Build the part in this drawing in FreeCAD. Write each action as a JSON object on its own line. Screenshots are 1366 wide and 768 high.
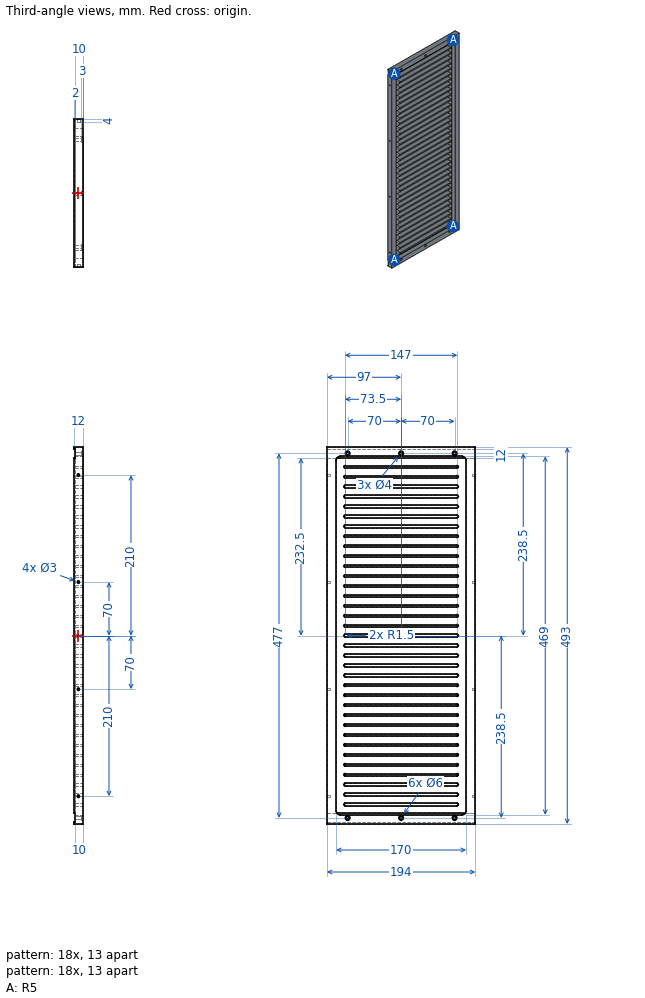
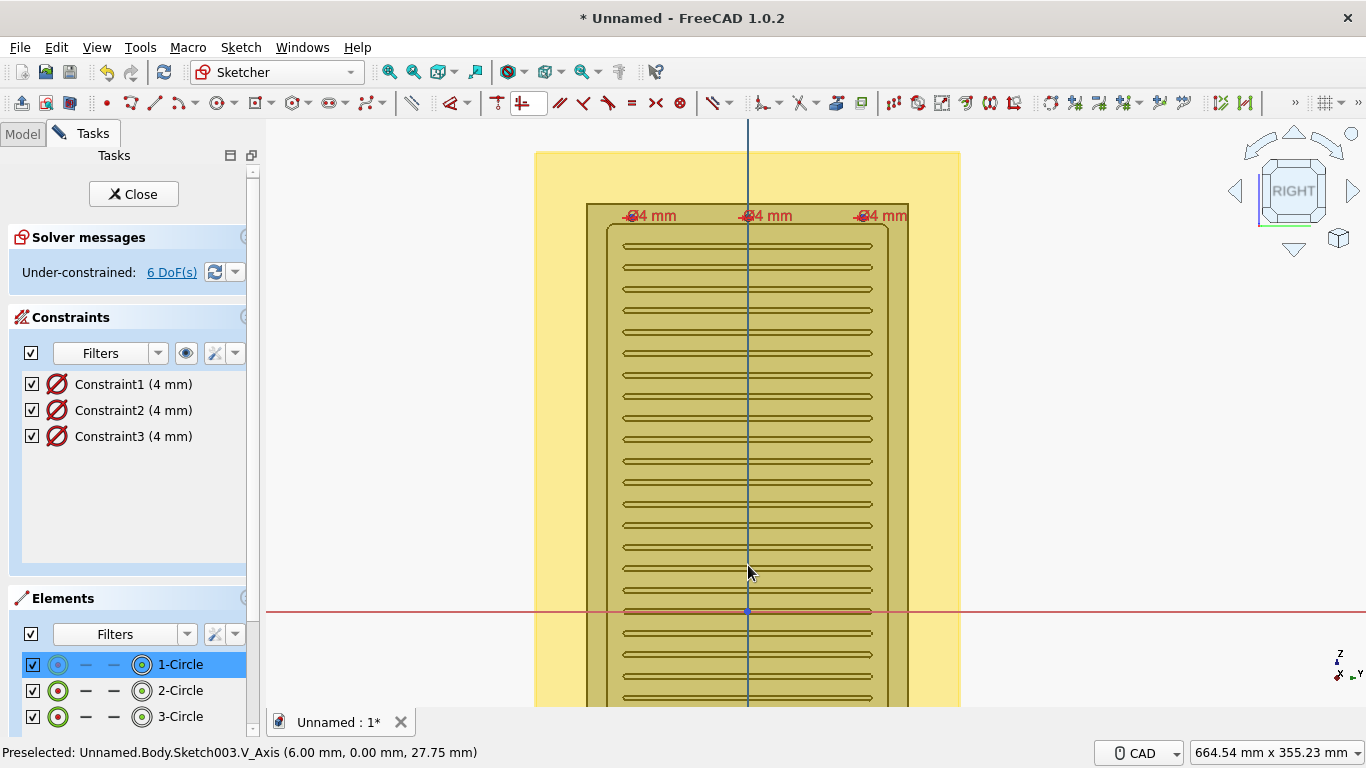
{"action": "left_click", "coordinate": [498, 104]}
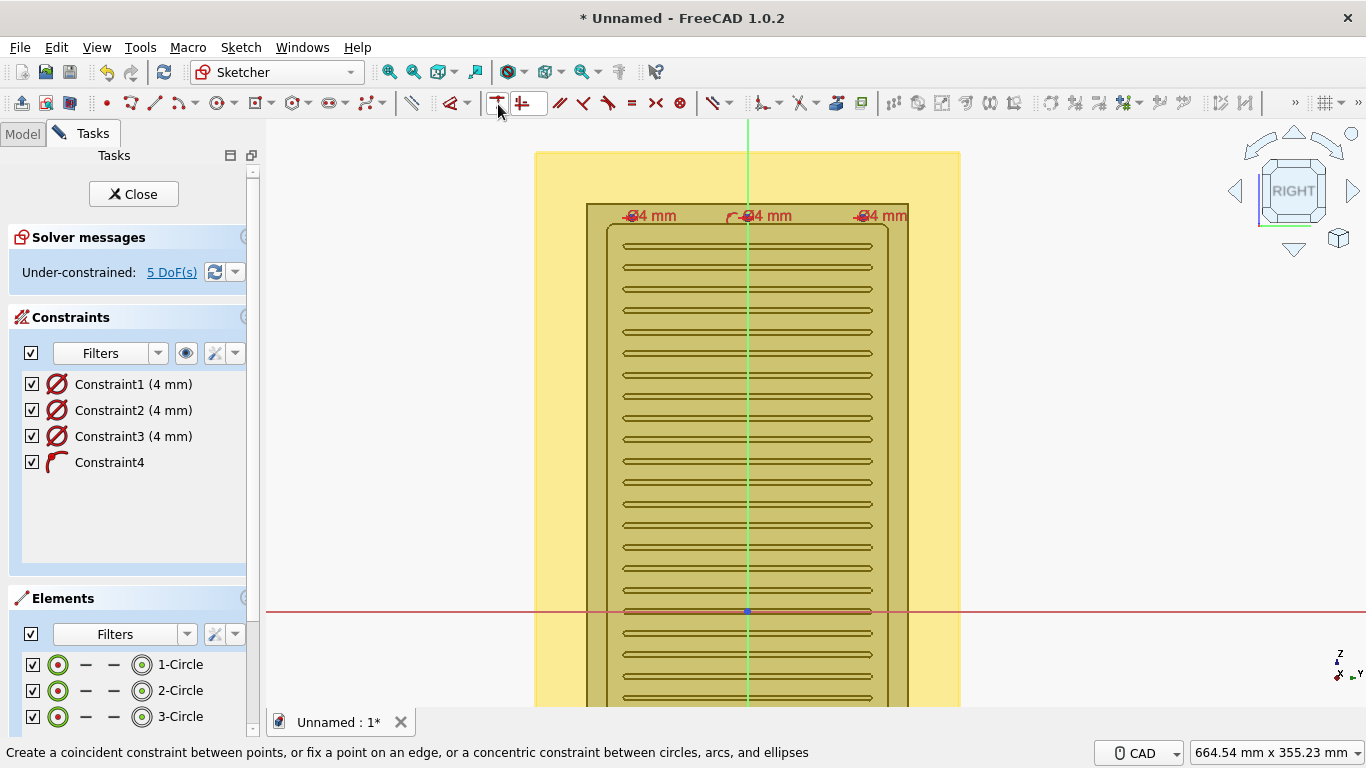
{"action": "left_click", "coordinate": [748, 218]}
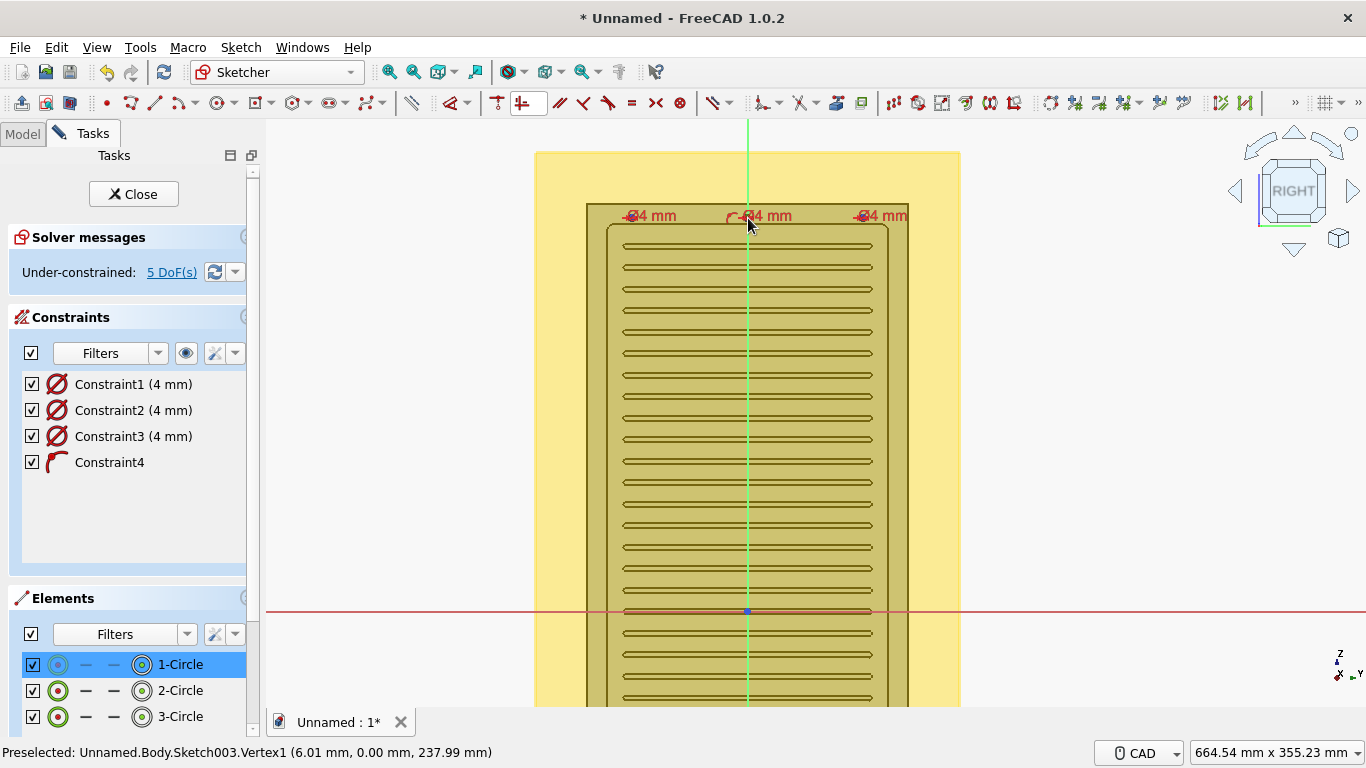
{"action": "left_click", "coordinate": [863, 218]}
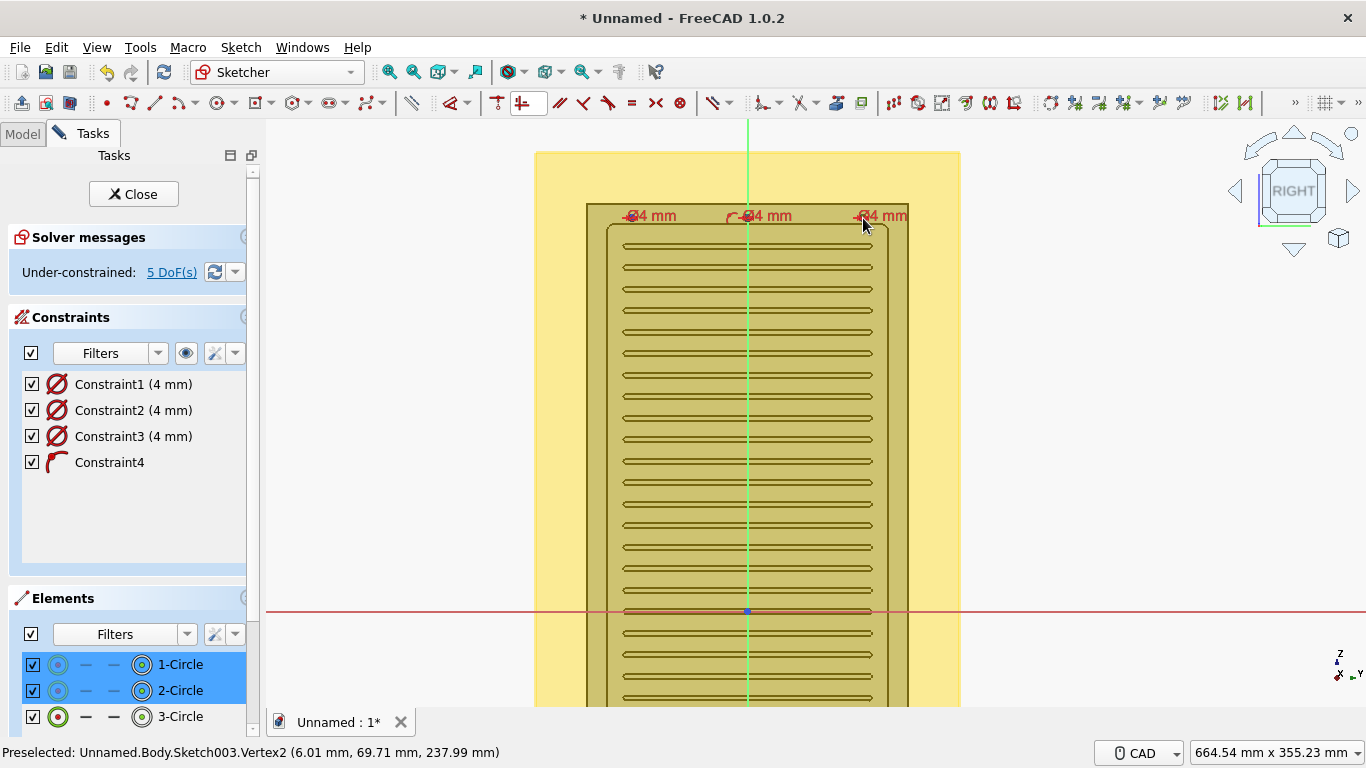
{"action": "left_click", "coordinate": [542, 104]}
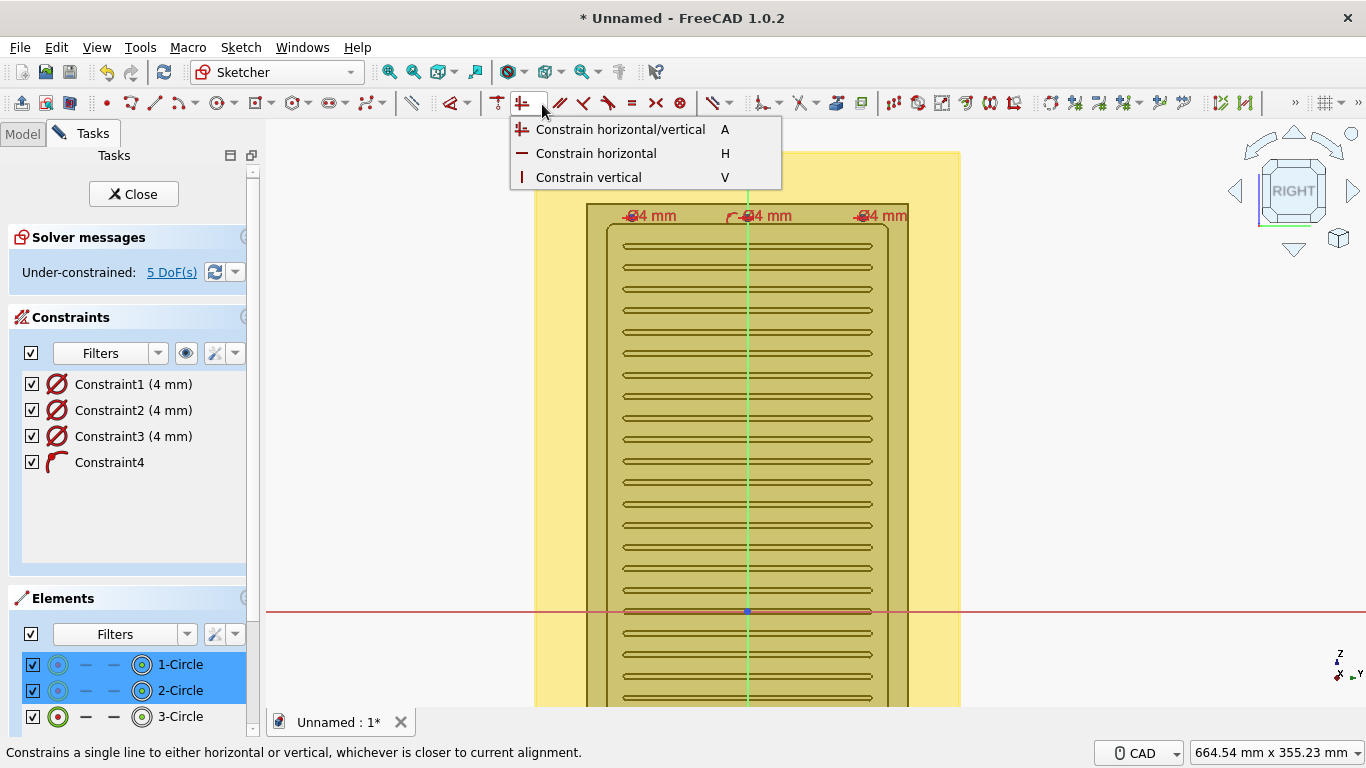
{"action": "left_click", "coordinate": [646, 153]}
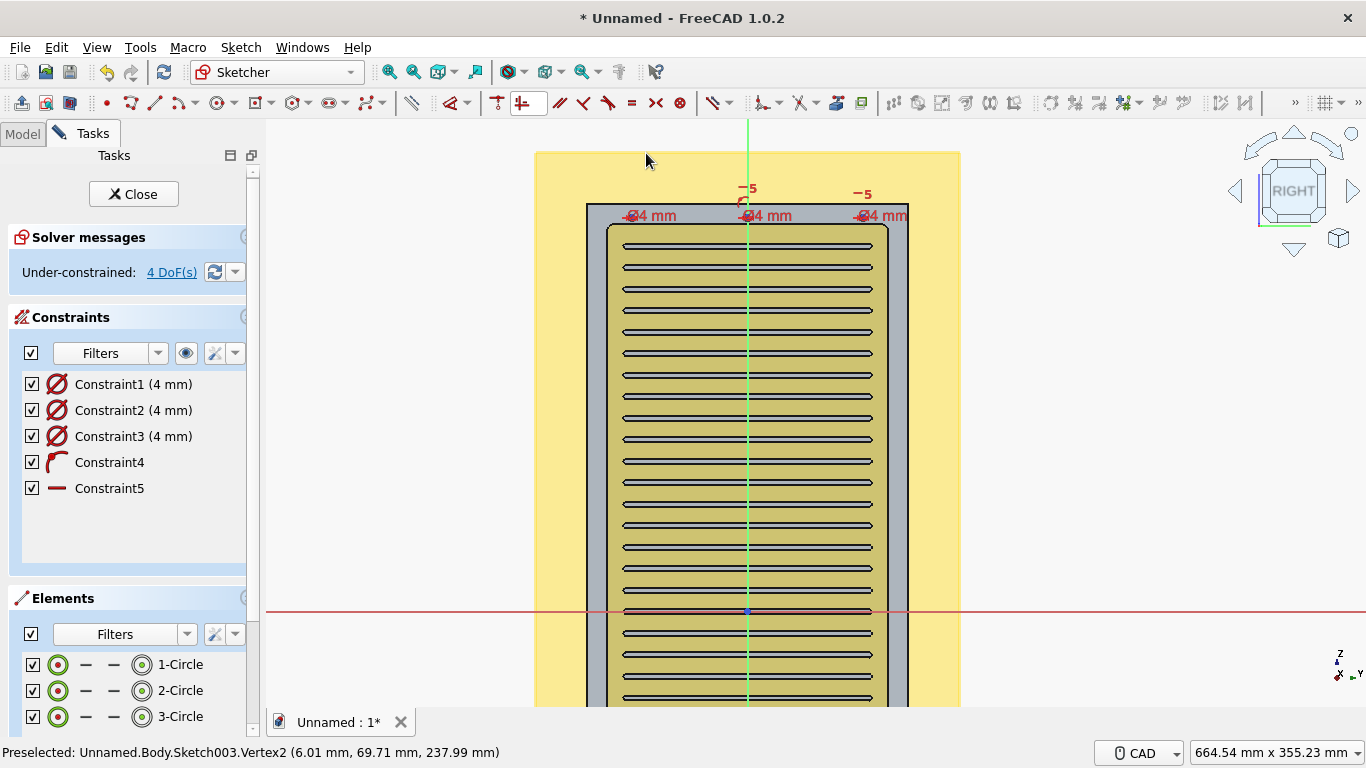
{"action": "left_click", "coordinate": [748, 218]}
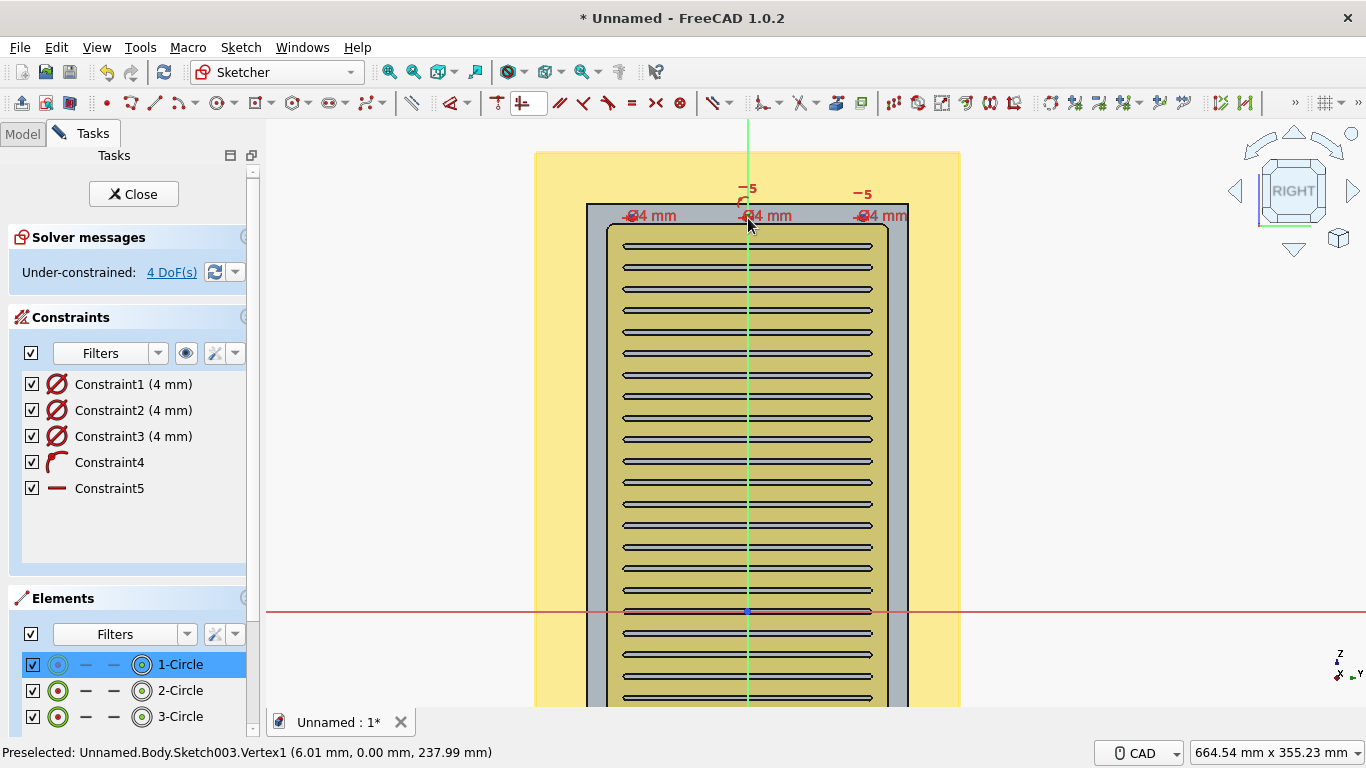
{"action": "left_click", "coordinate": [632, 218]}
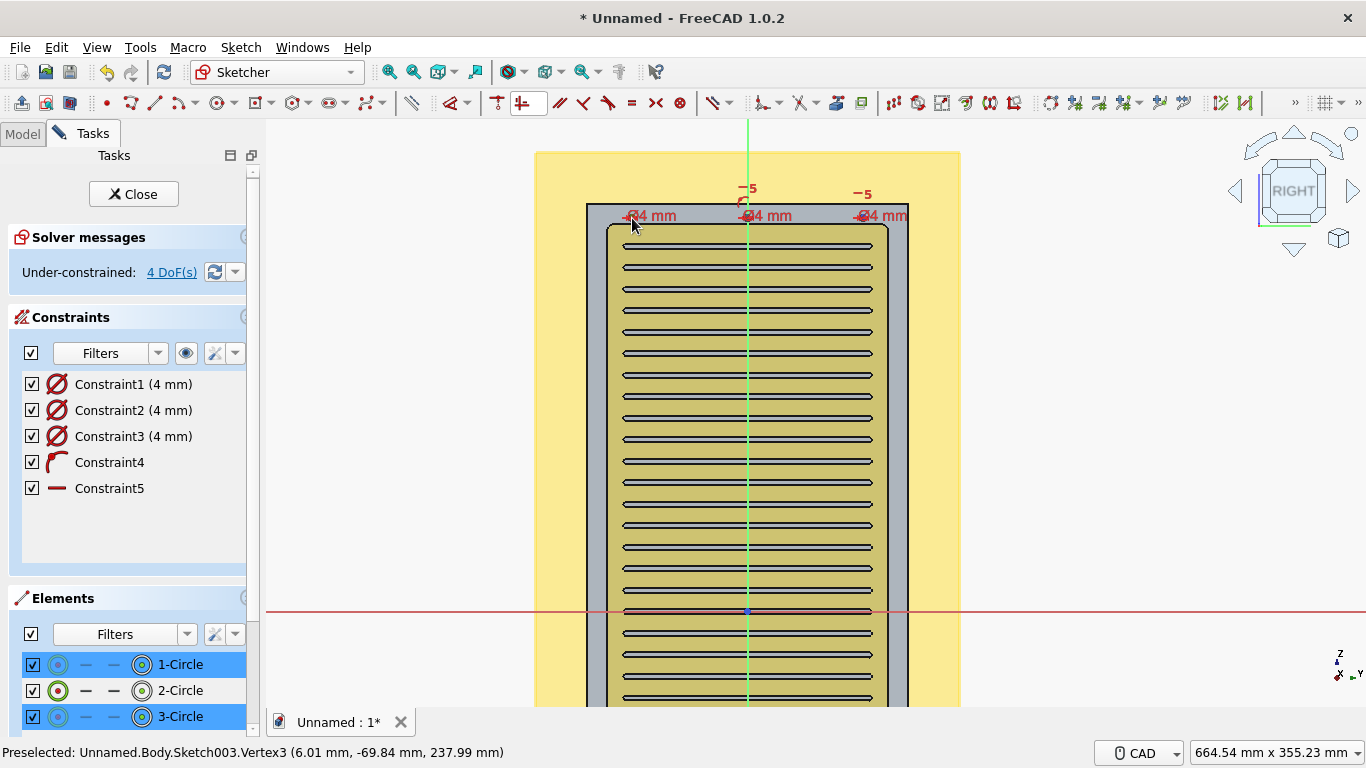
{"action": "left_click", "coordinate": [542, 104]}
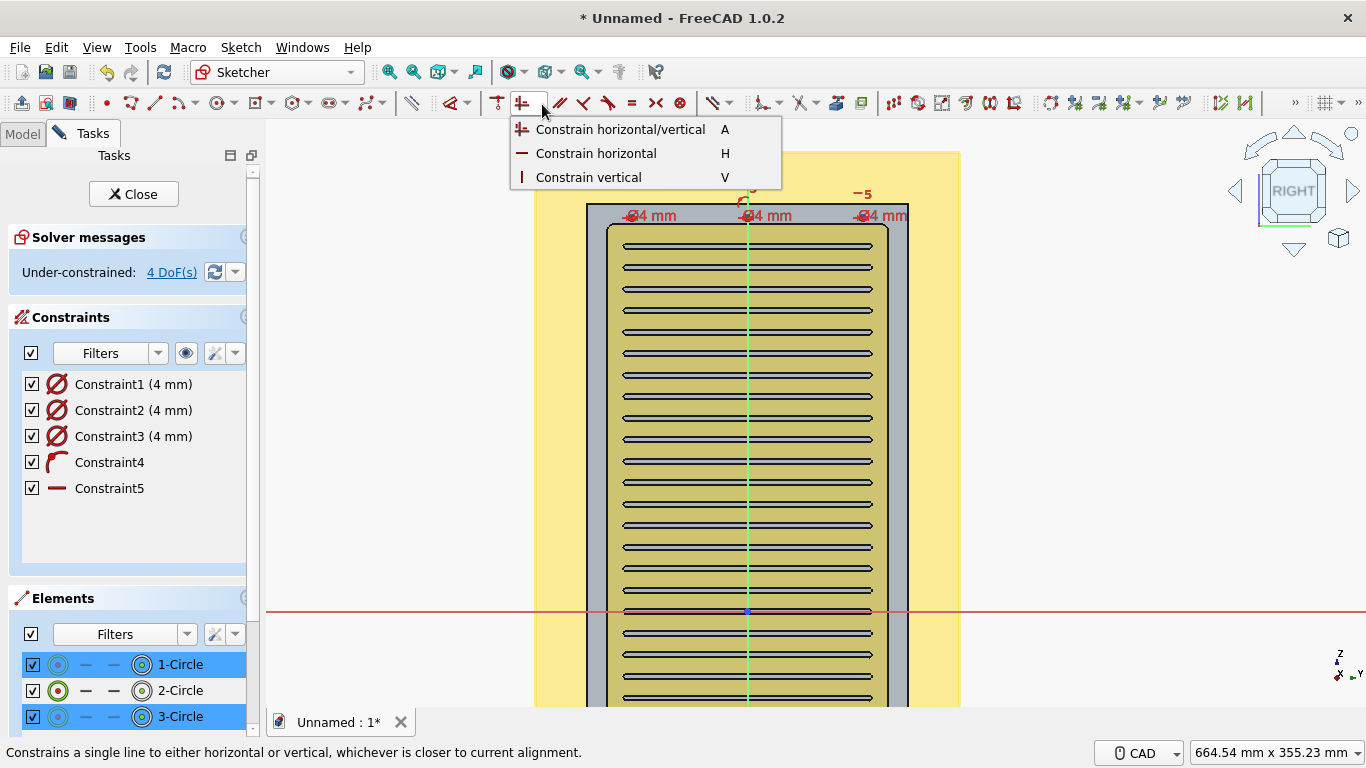
{"action": "left_click", "coordinate": [646, 153]}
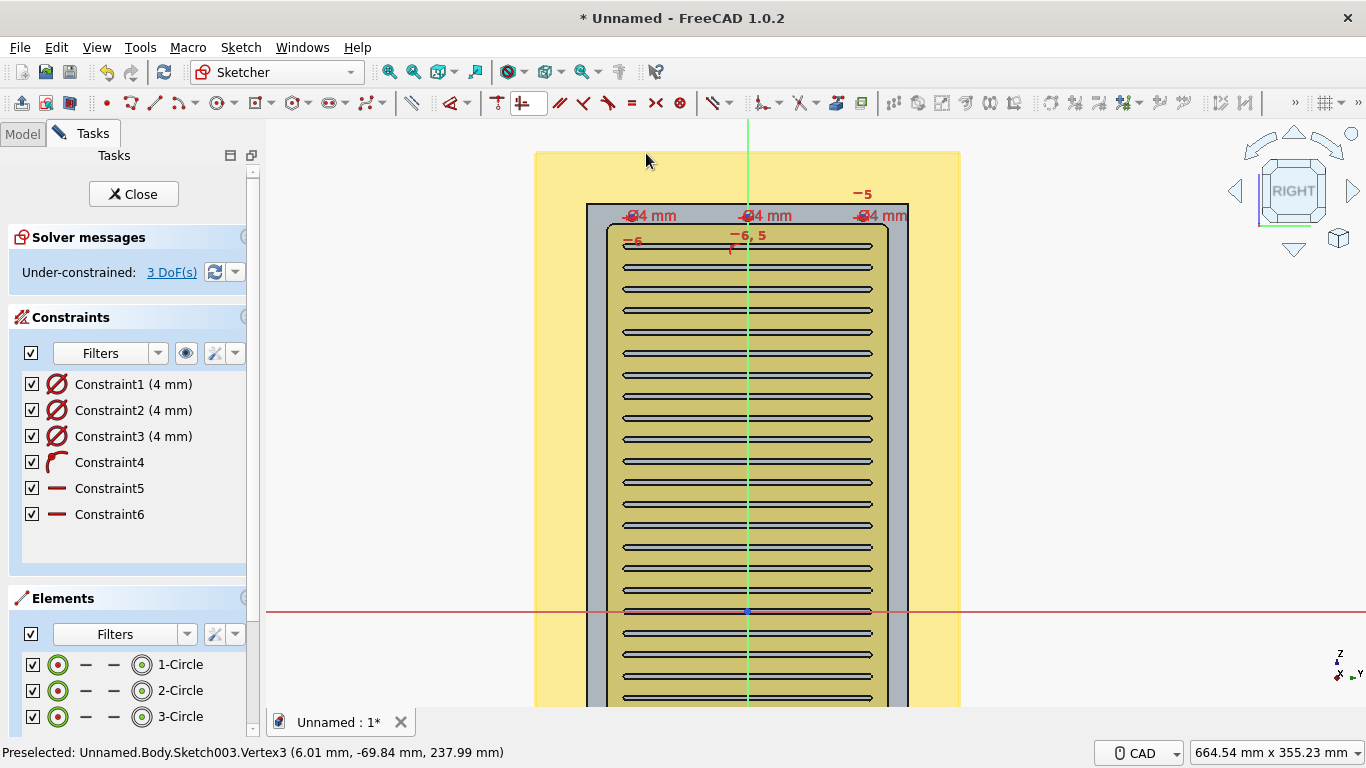
{"action": "left_click", "coordinate": [863, 218]}